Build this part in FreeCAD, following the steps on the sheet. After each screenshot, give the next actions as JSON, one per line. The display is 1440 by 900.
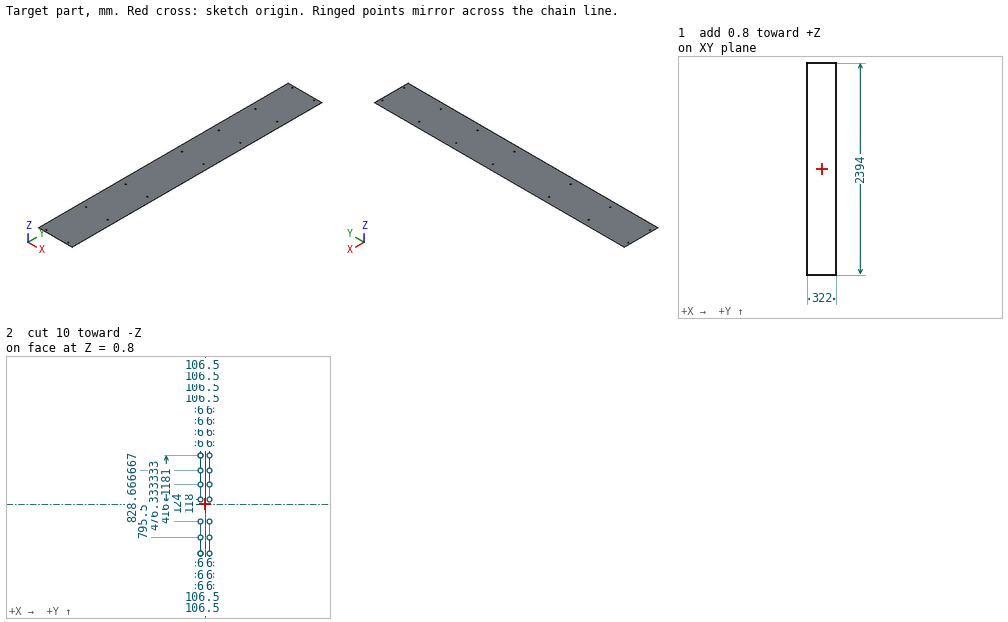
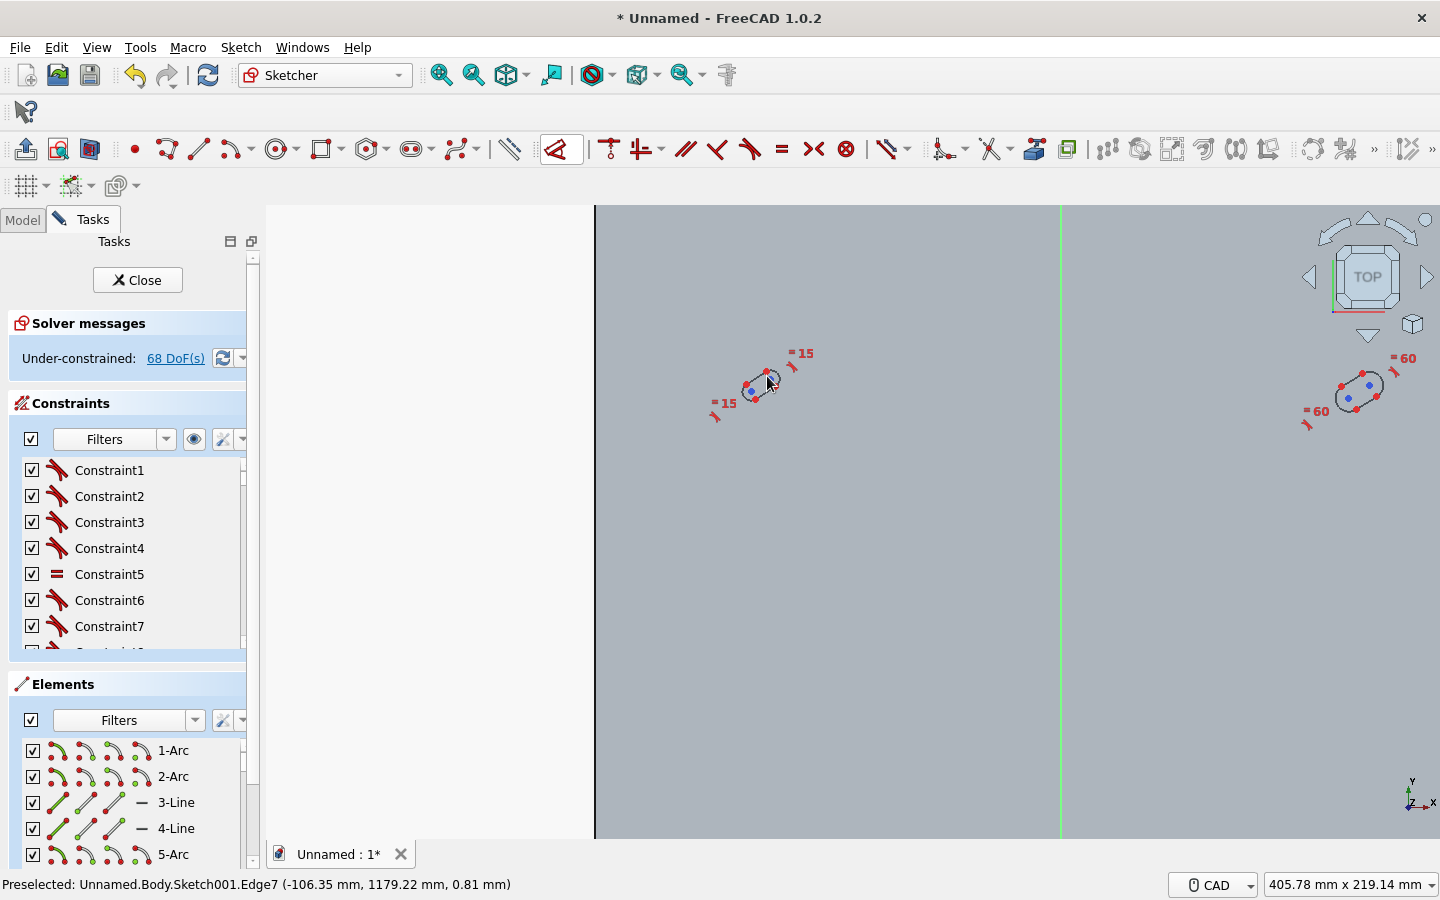
{"action": "left_click", "coordinate": [754, 379]}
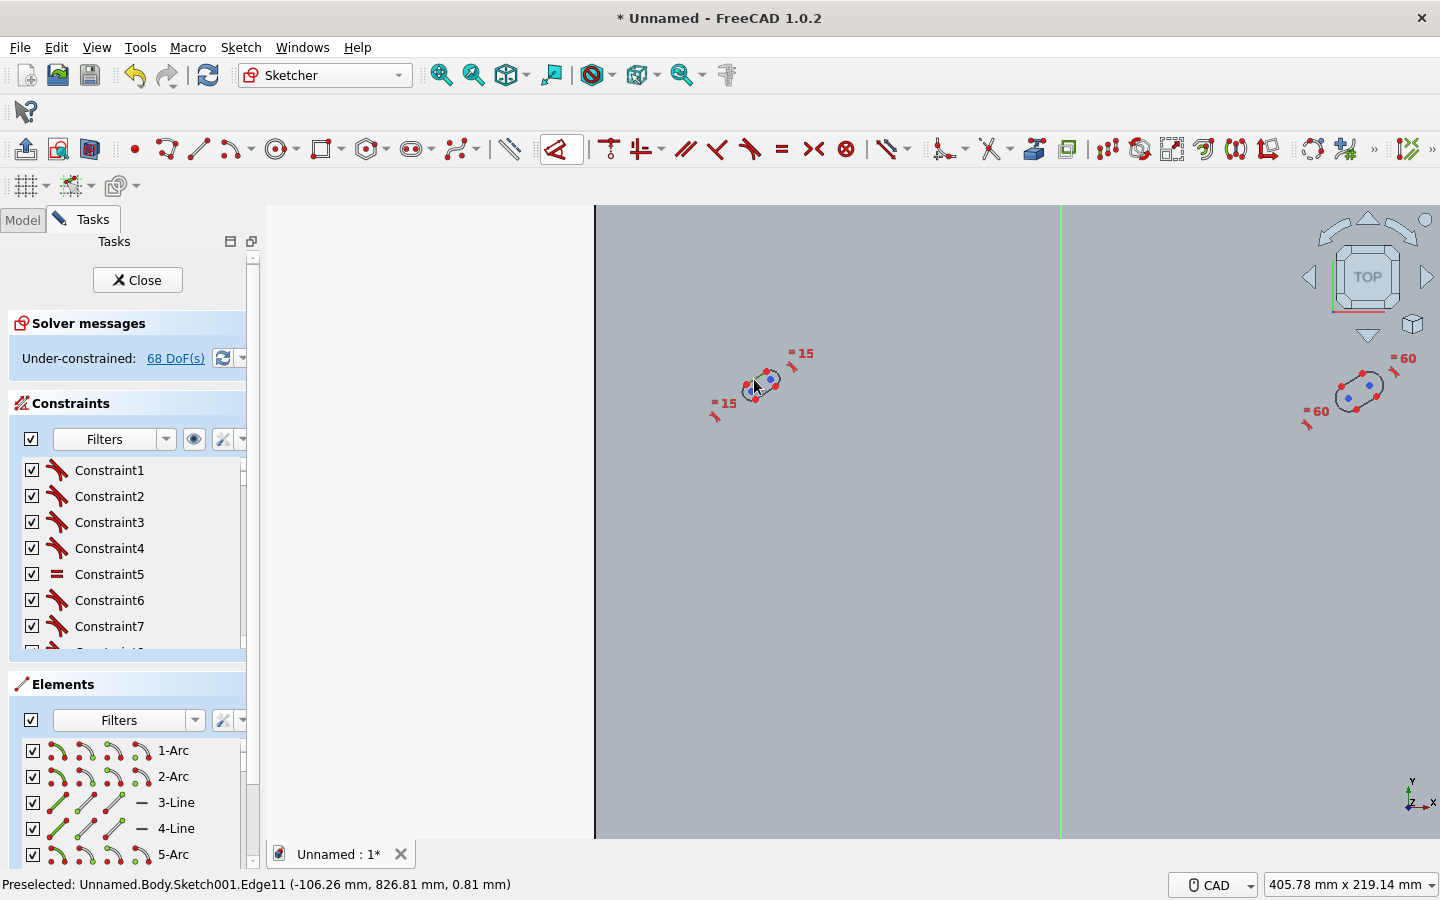
{"action": "left_click", "coordinate": [664, 150]}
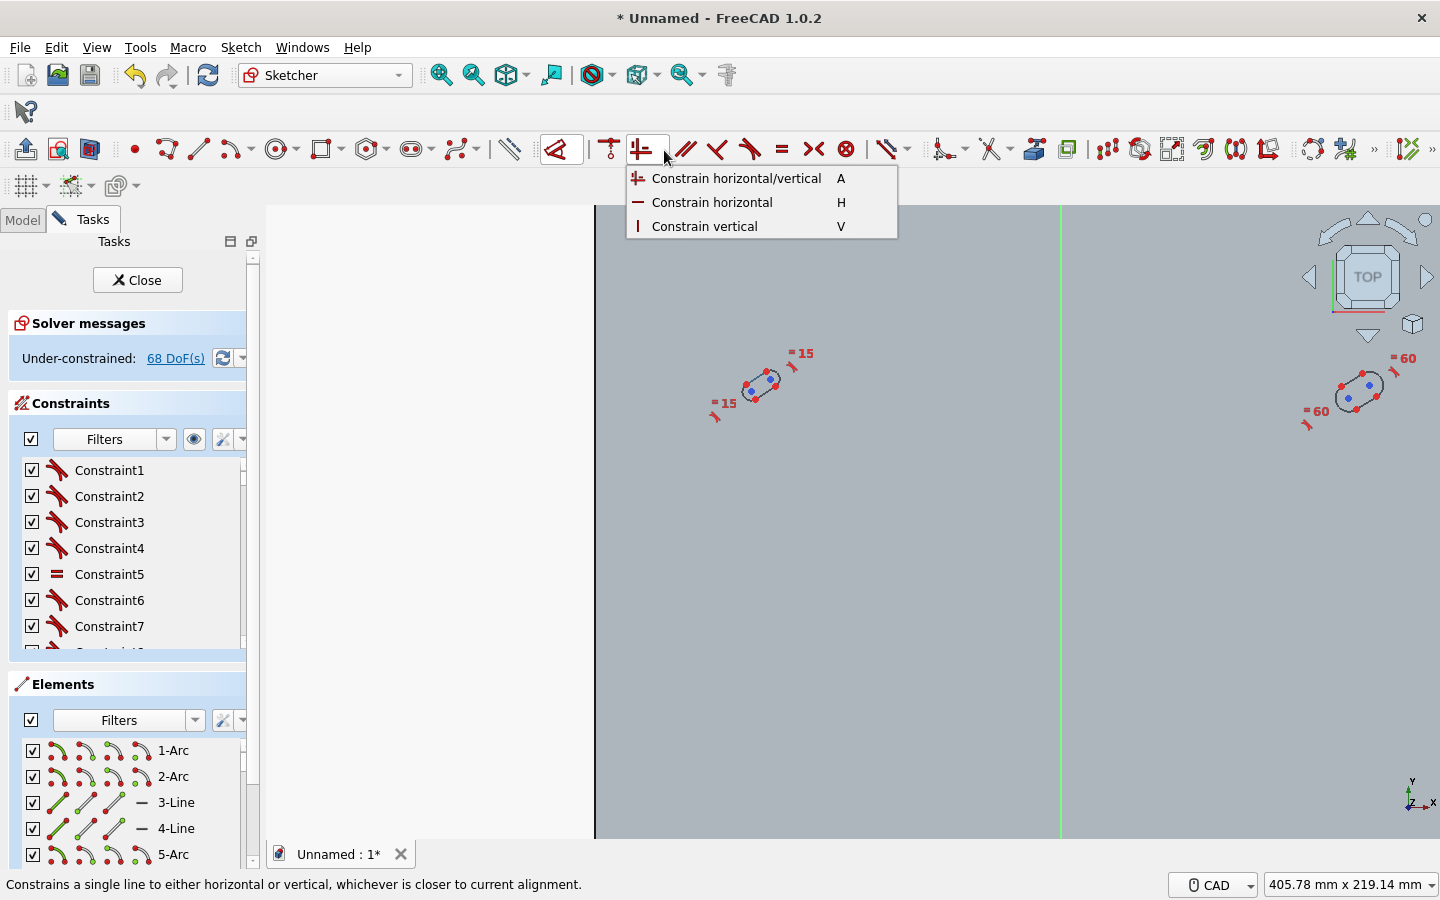
{"action": "left_click", "coordinate": [762, 202]}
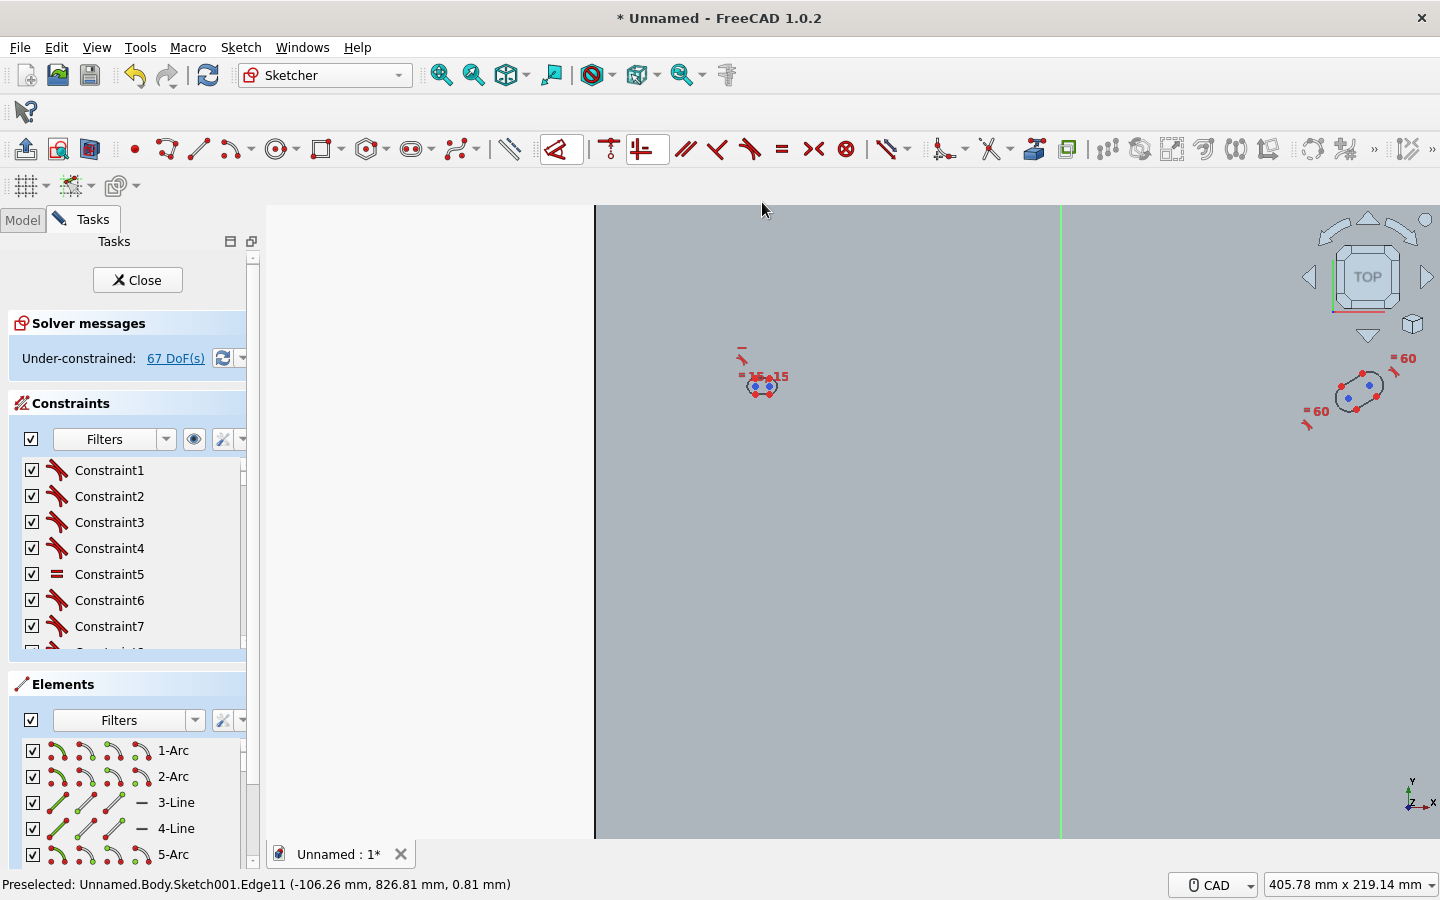
{"action": "scroll", "coordinate": [767, 376], "scroll_direction": "down", "scroll_amount": 14}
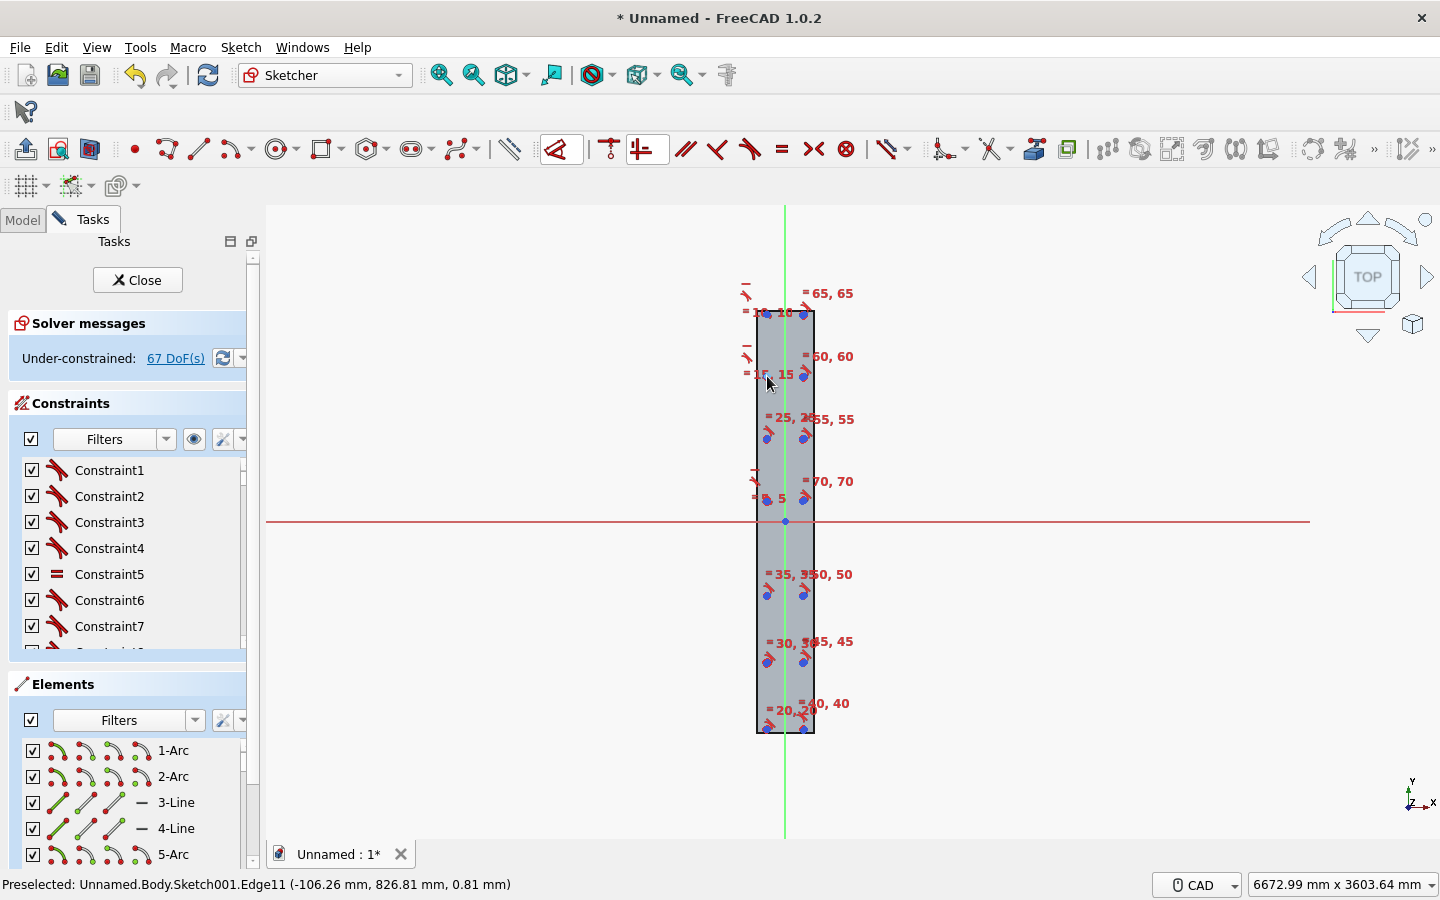
{"action": "scroll", "coordinate": [766, 729], "scroll_direction": "up", "scroll_amount": 14}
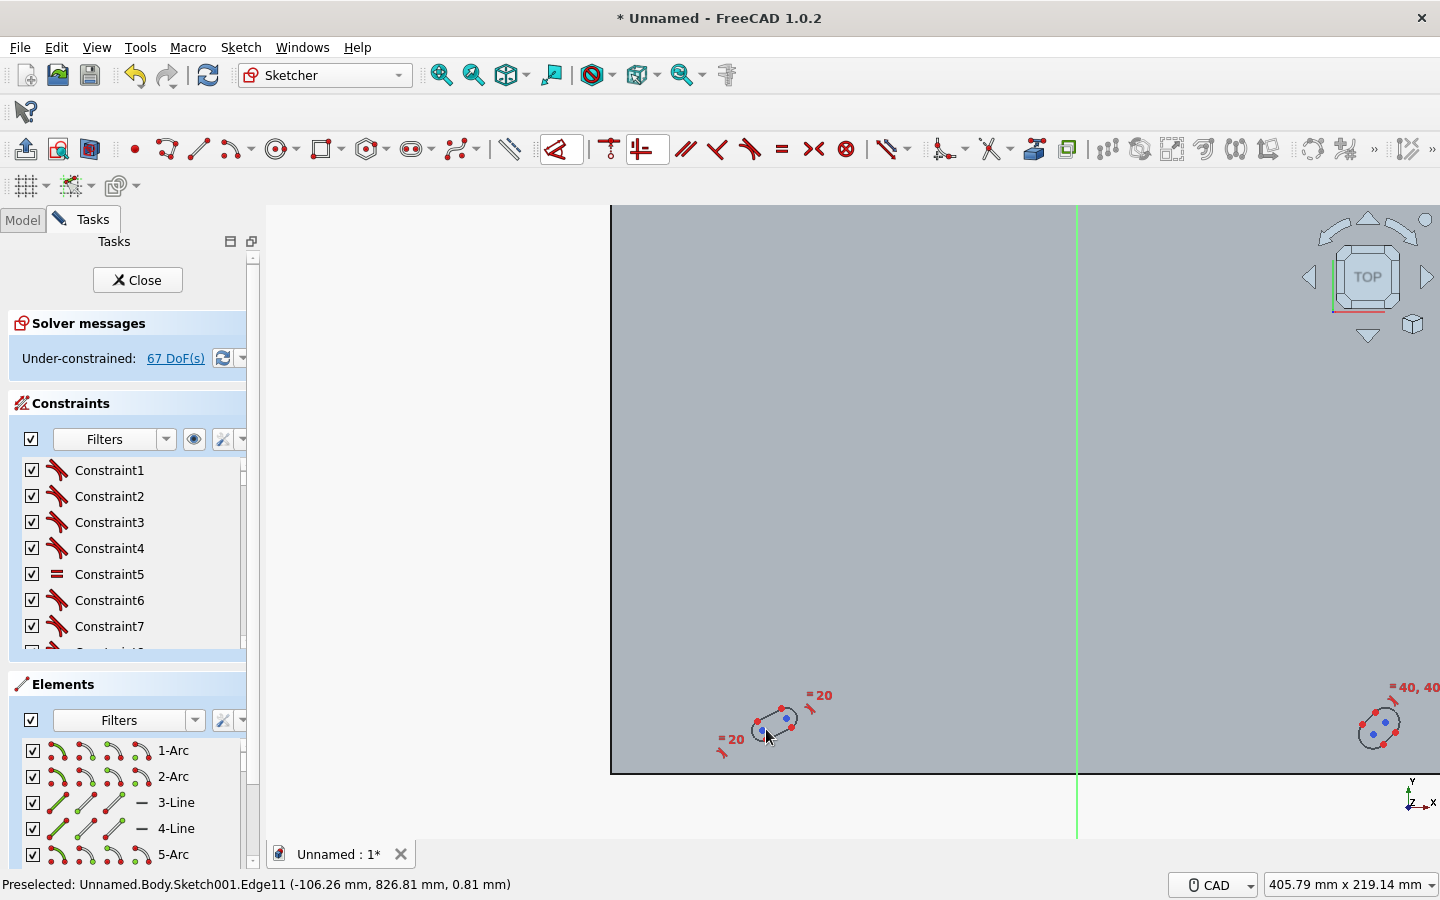
{"action": "left_click", "coordinate": [767, 716]}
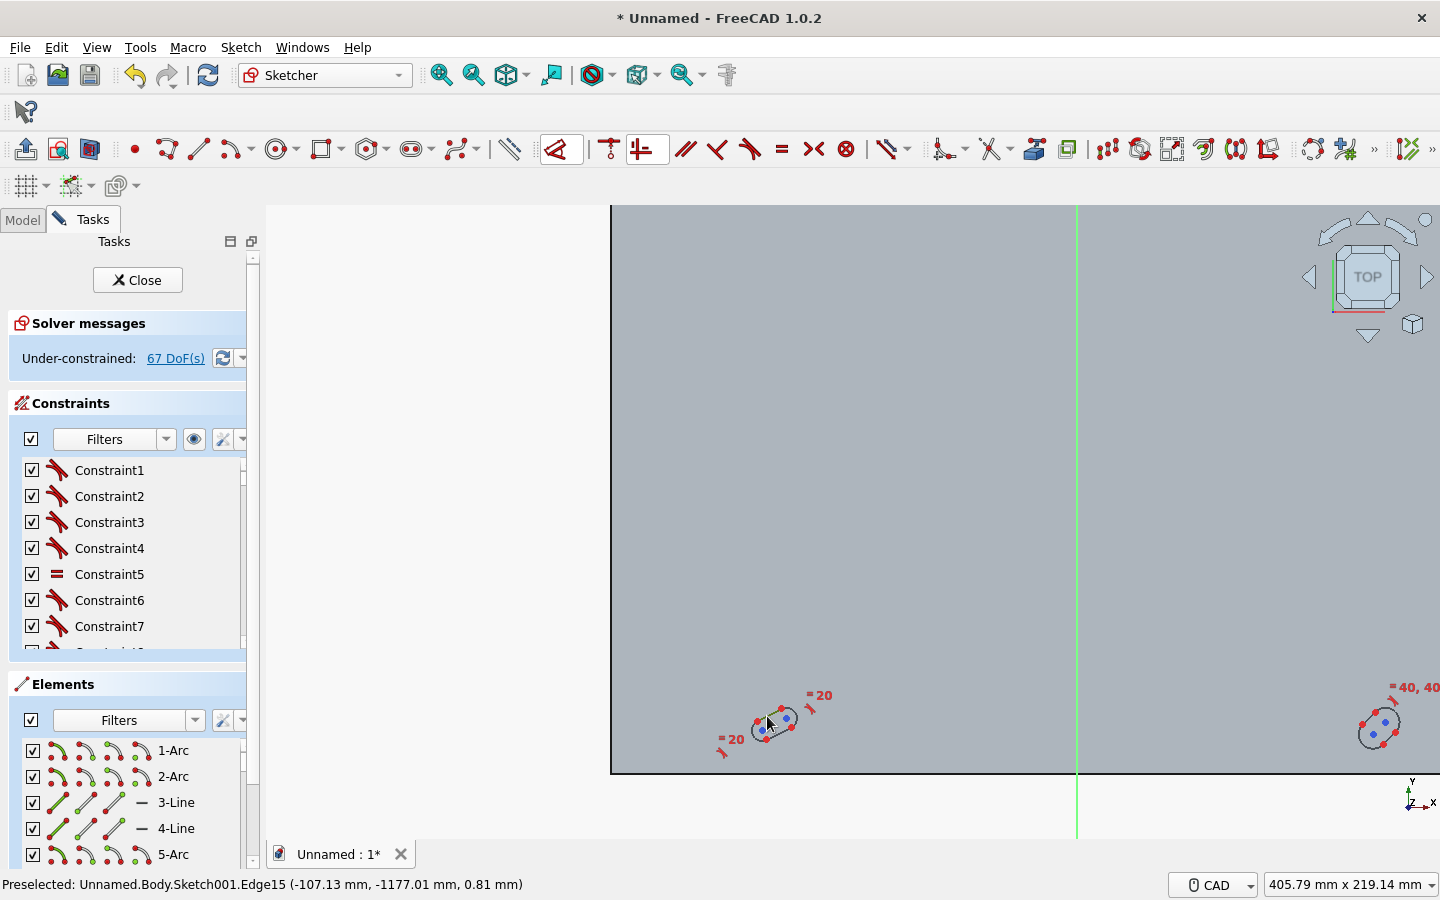
{"action": "key", "text": "h"}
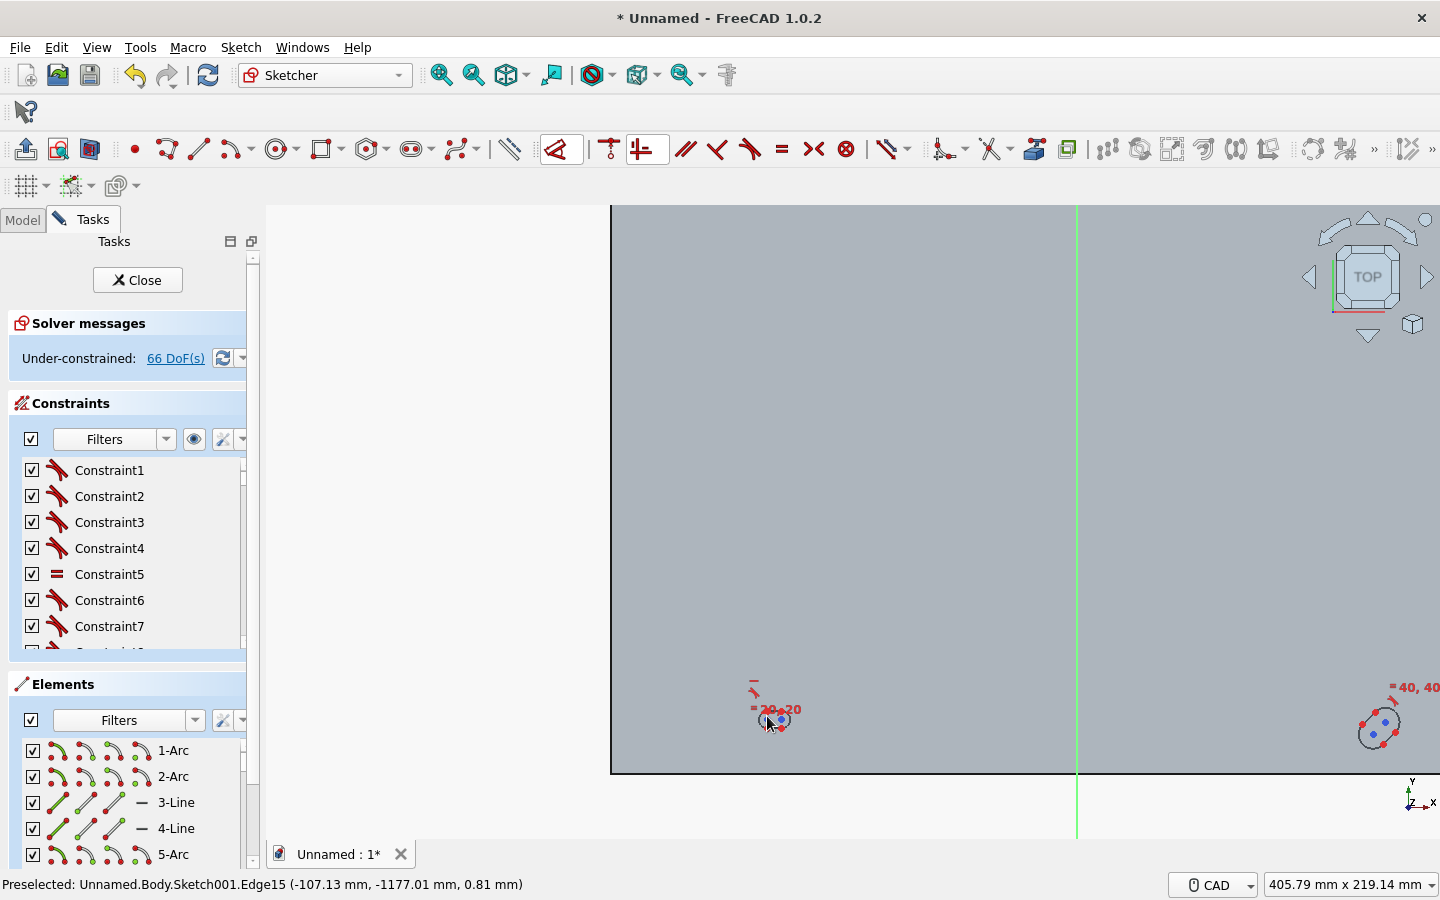
{"action": "scroll", "coordinate": [766, 730], "scroll_direction": "down", "scroll_amount": 14}